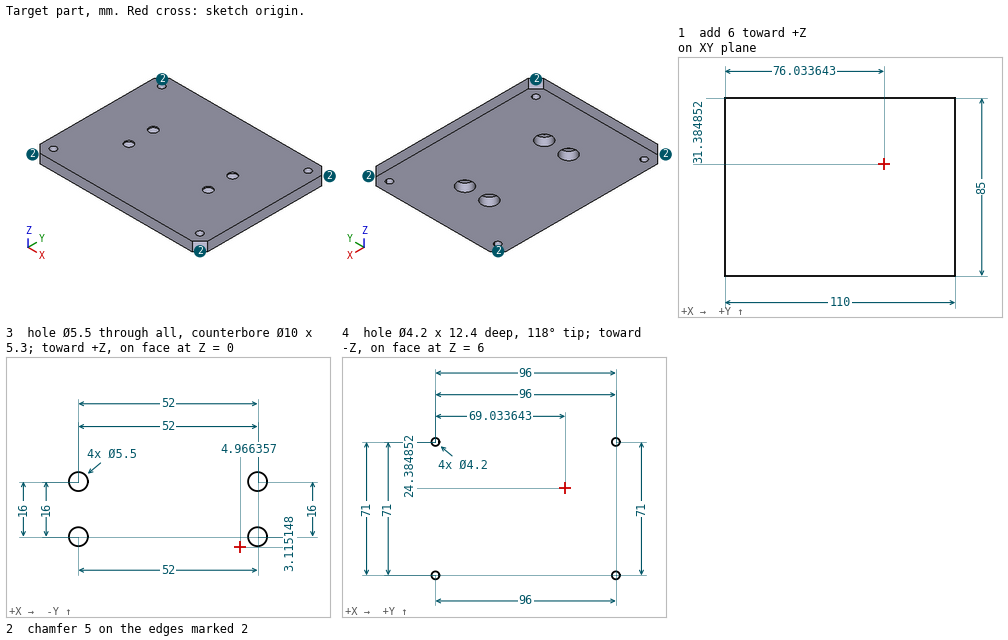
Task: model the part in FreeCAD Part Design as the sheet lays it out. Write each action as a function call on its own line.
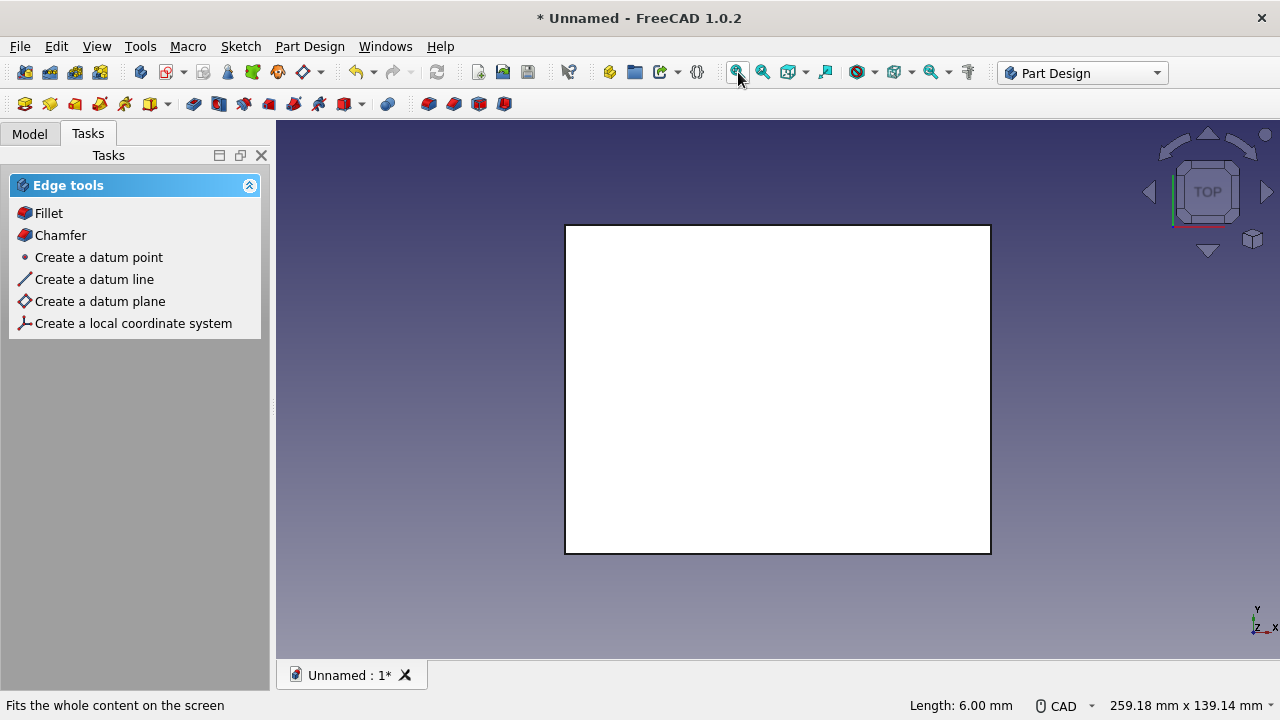
key(1)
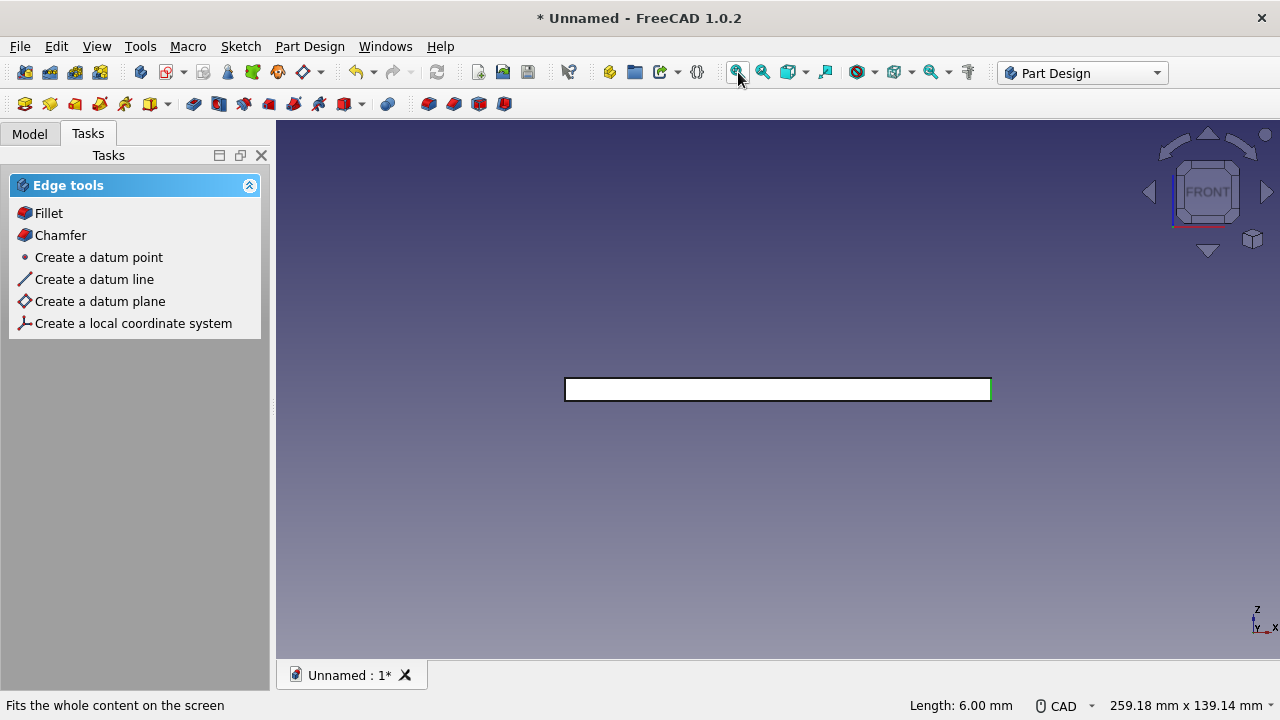
click(738, 72)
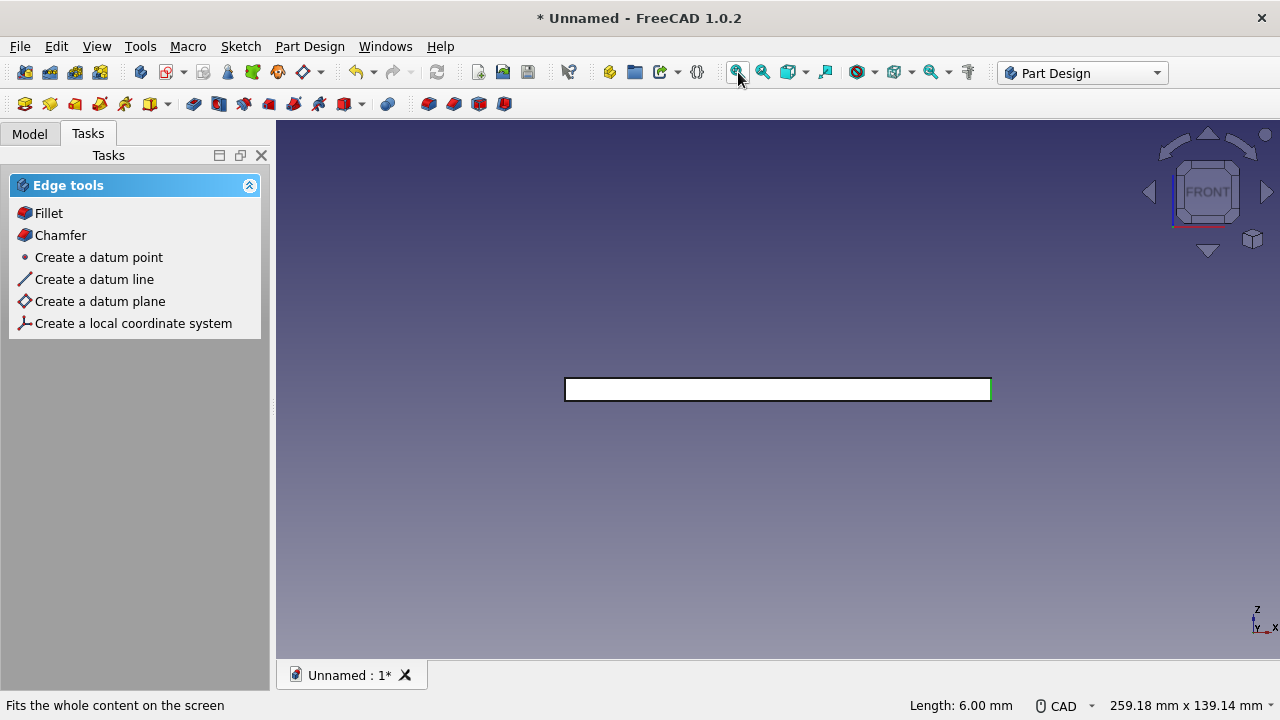
click(565, 389, ctrl)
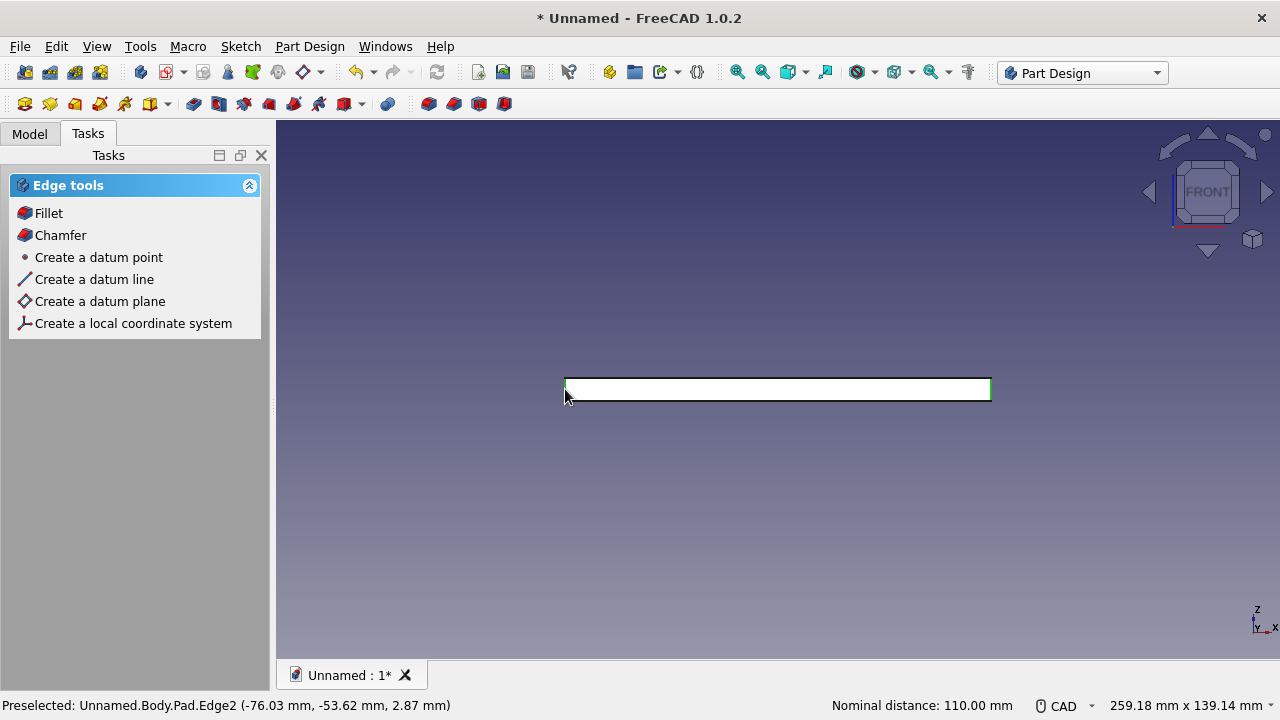
key(3)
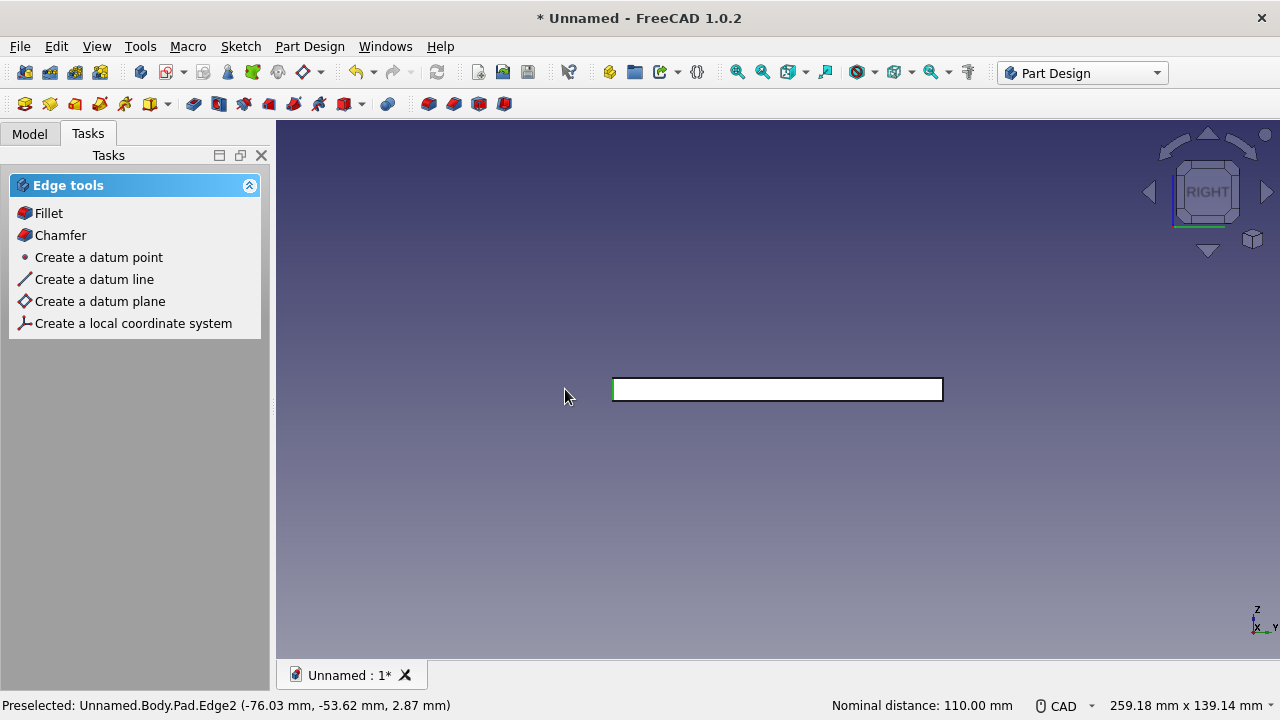
key(v)
key(f)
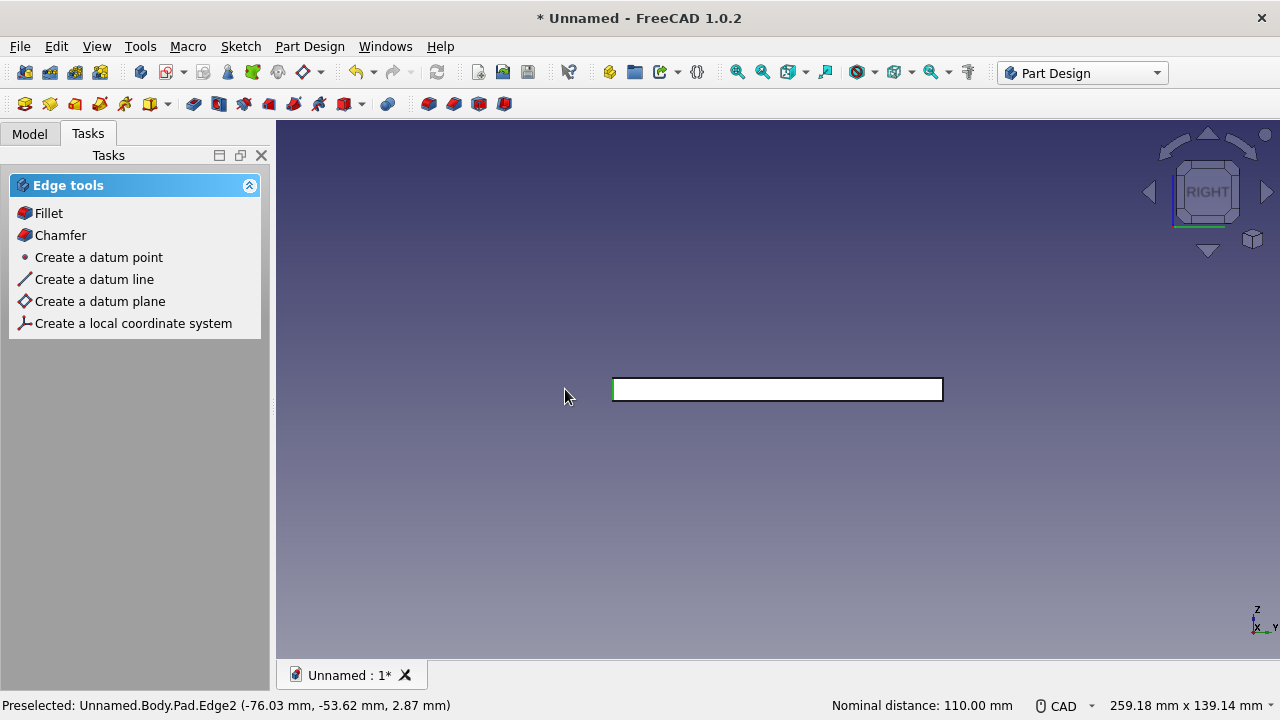
click(943, 388, ctrl)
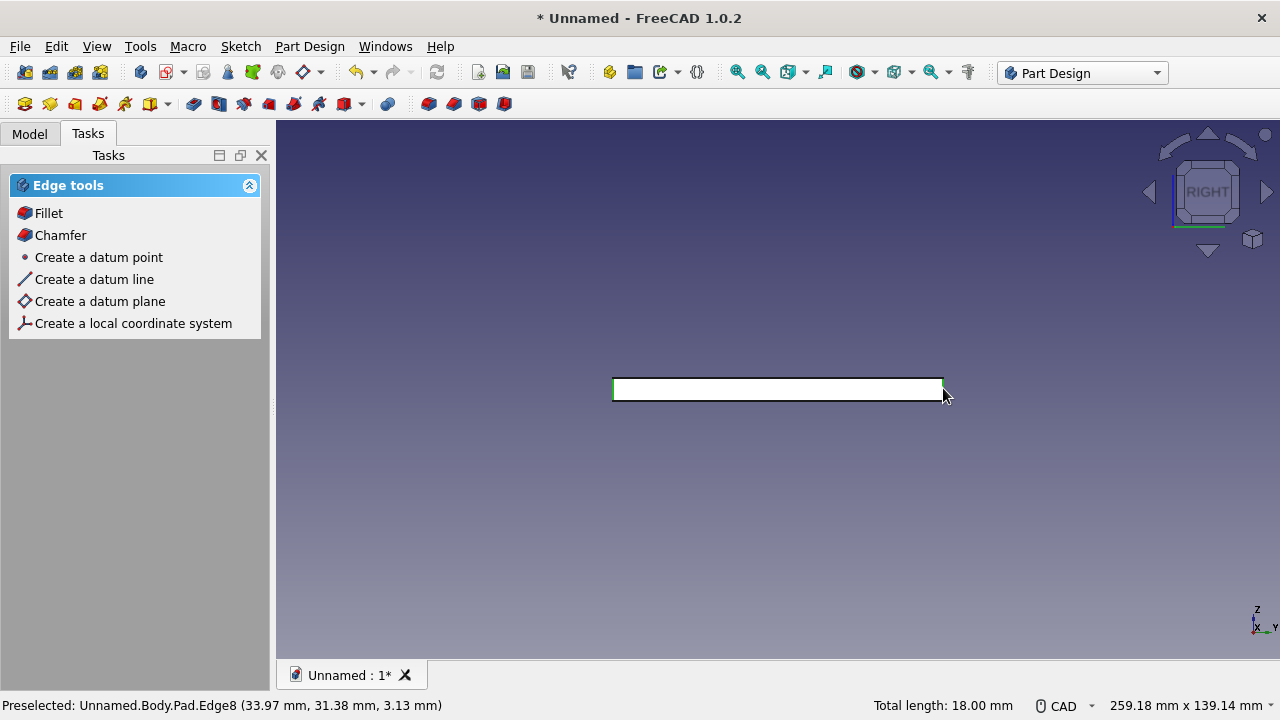
key(5)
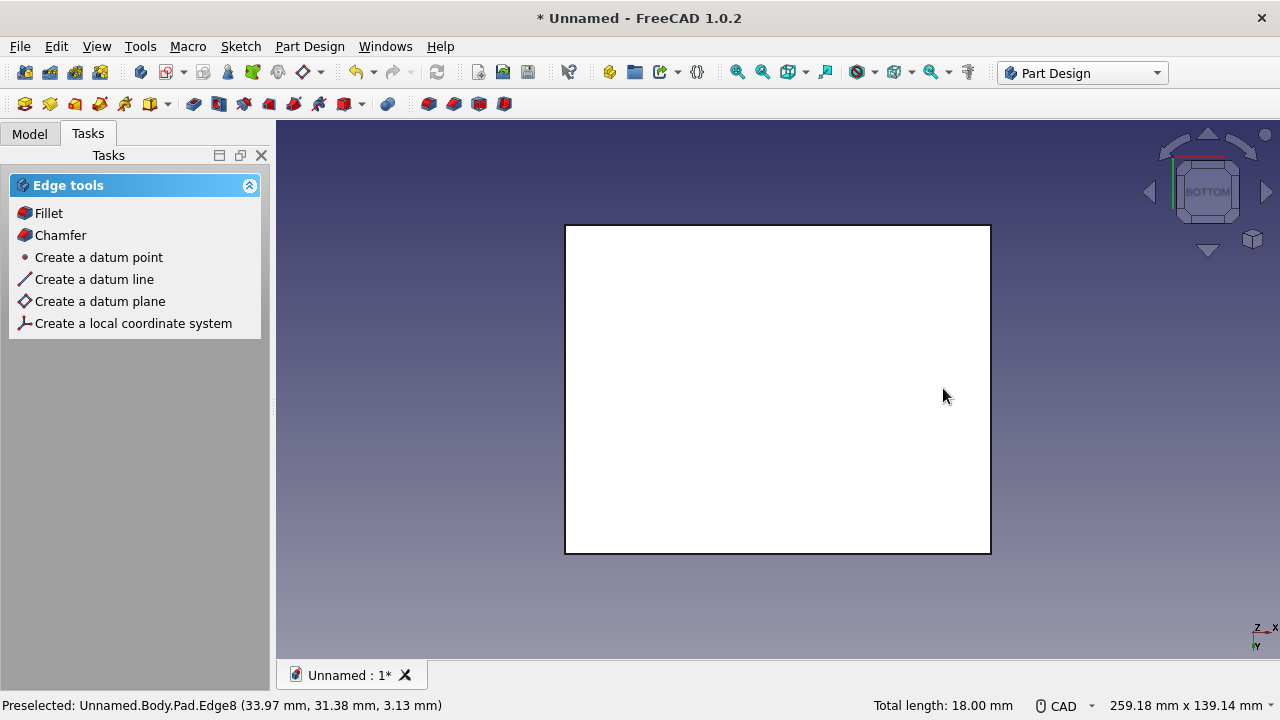
key(4)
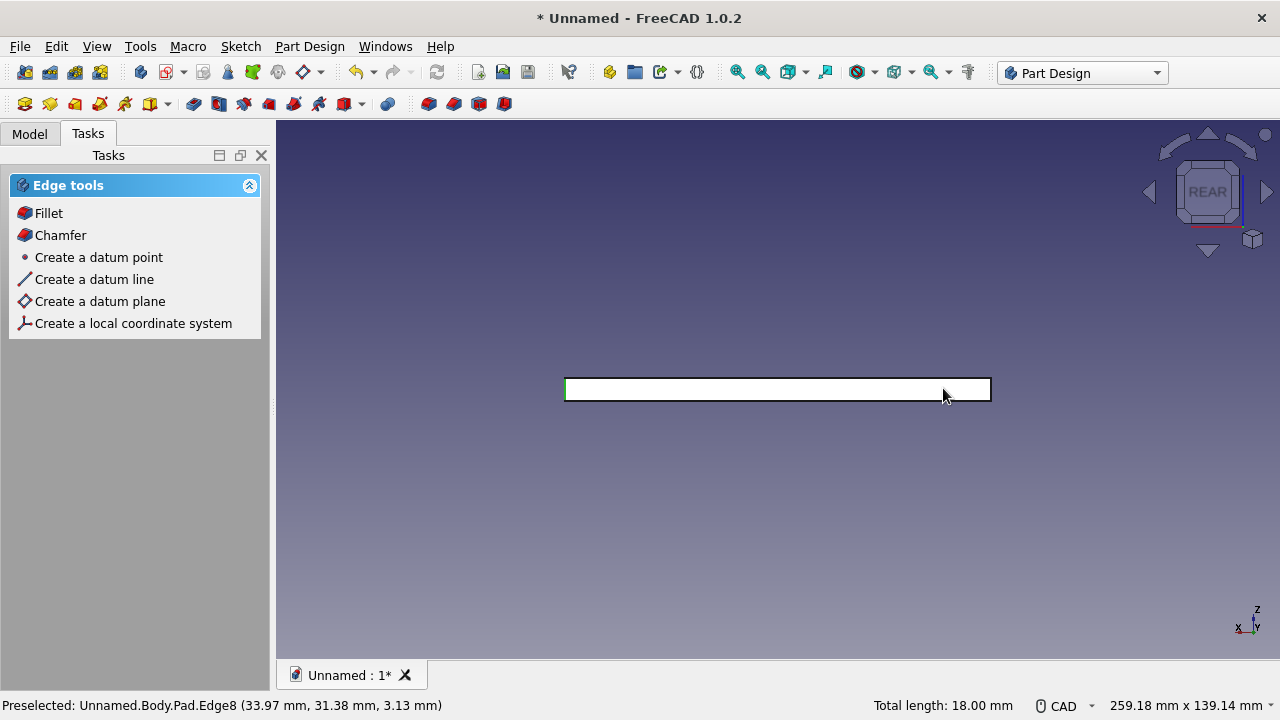
key(v)
key(f)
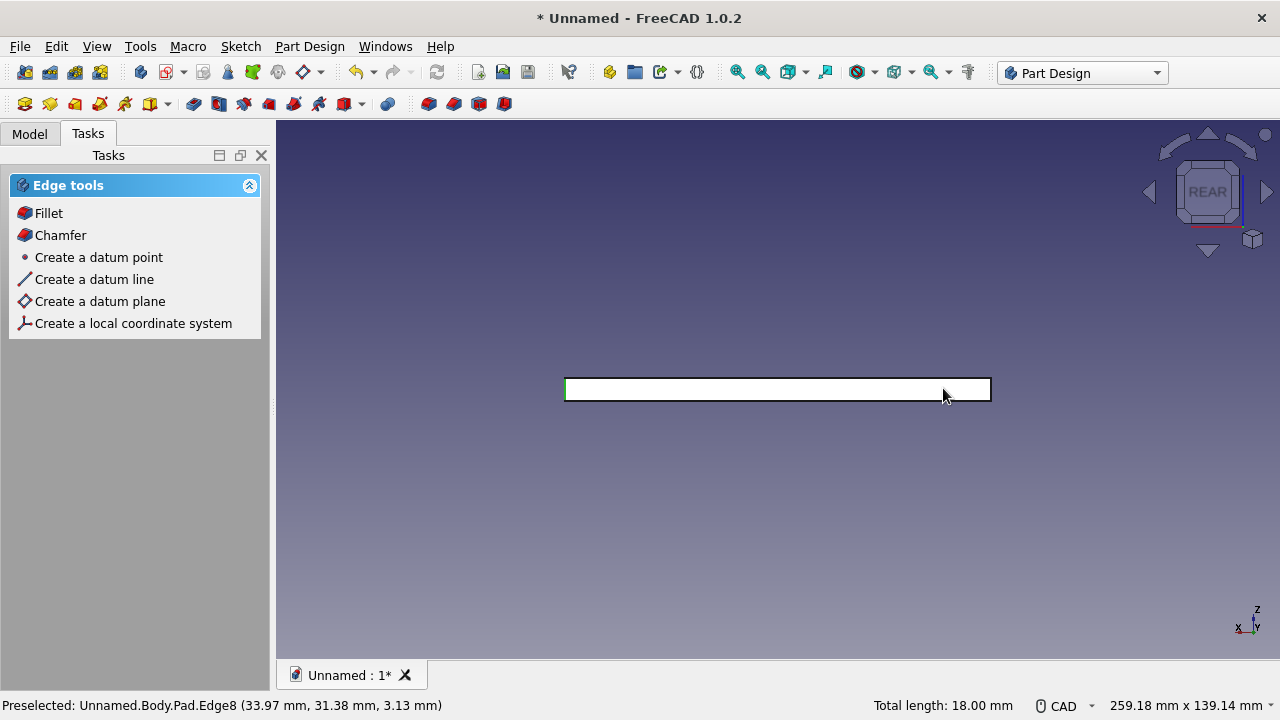
click(991, 389, ctrl)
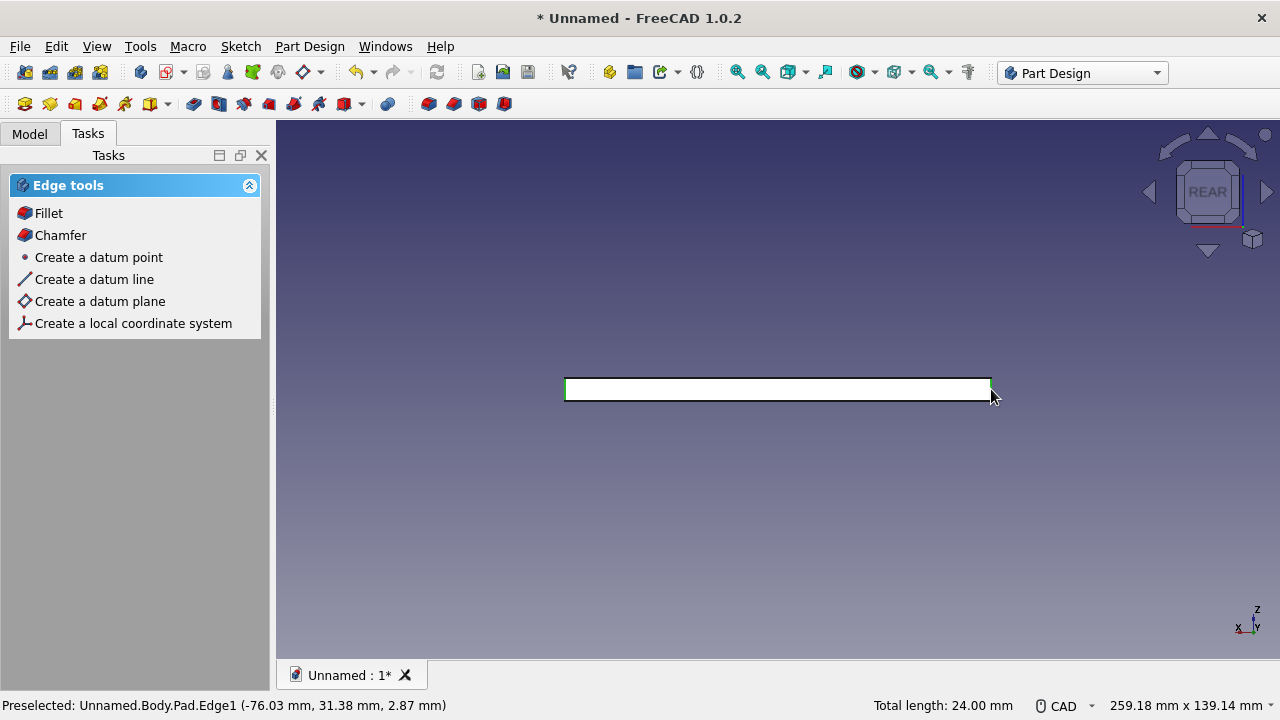
click(454, 104)